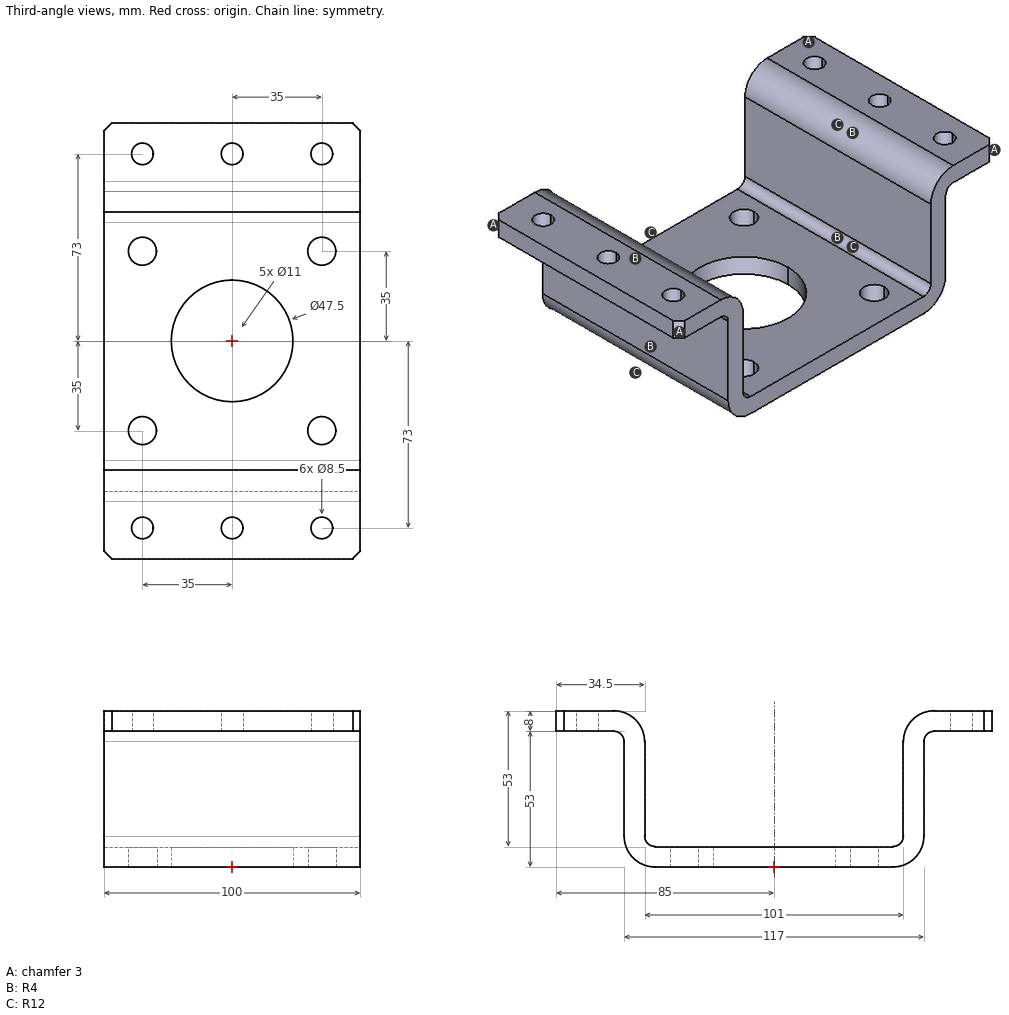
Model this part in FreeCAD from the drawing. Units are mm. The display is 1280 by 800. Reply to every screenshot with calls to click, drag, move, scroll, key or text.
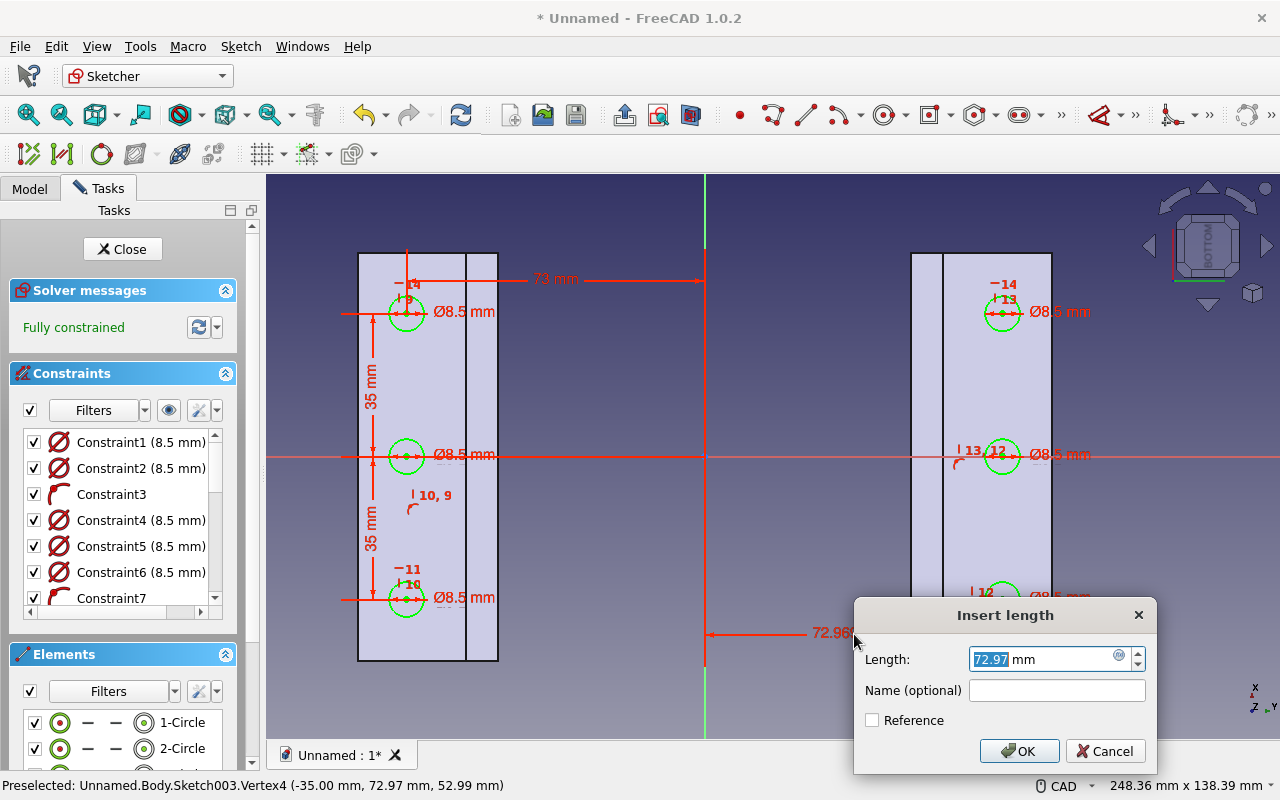
text(73)
key(Return)
key(Escape)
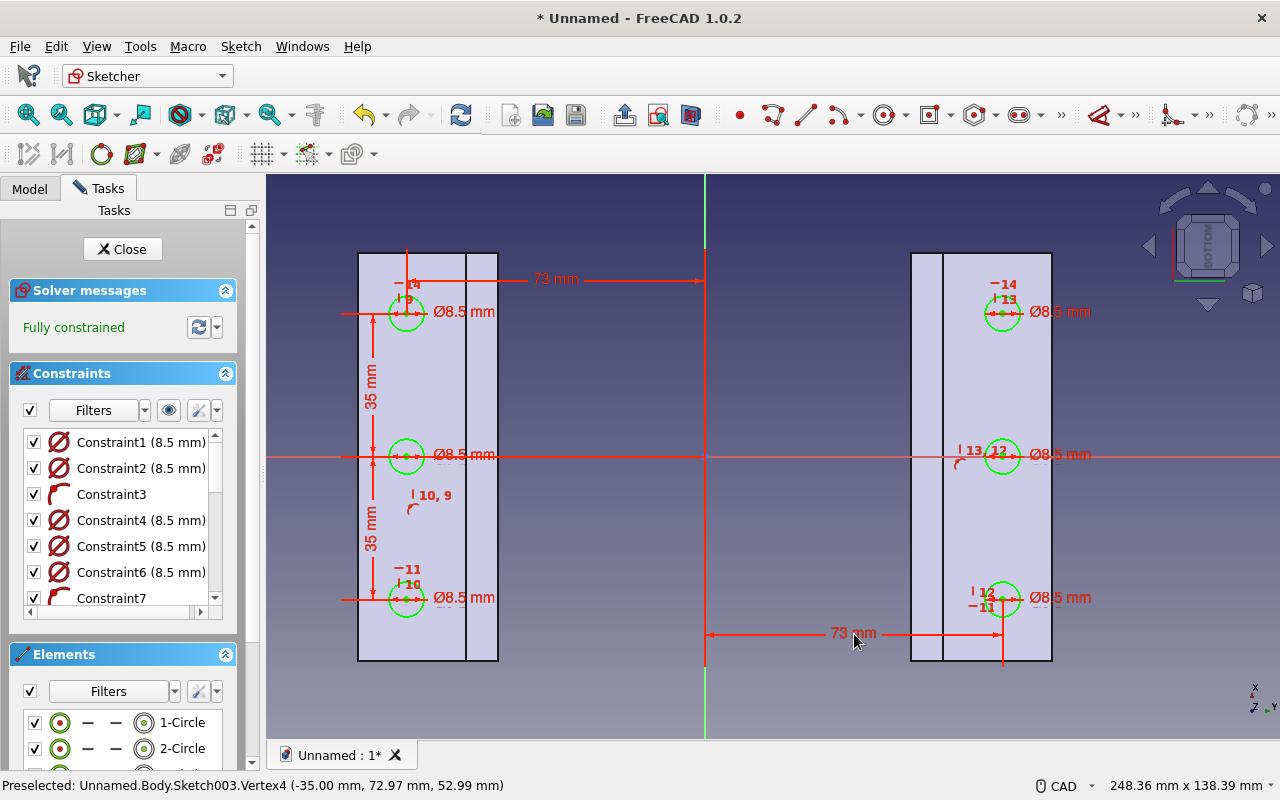
click(123, 249)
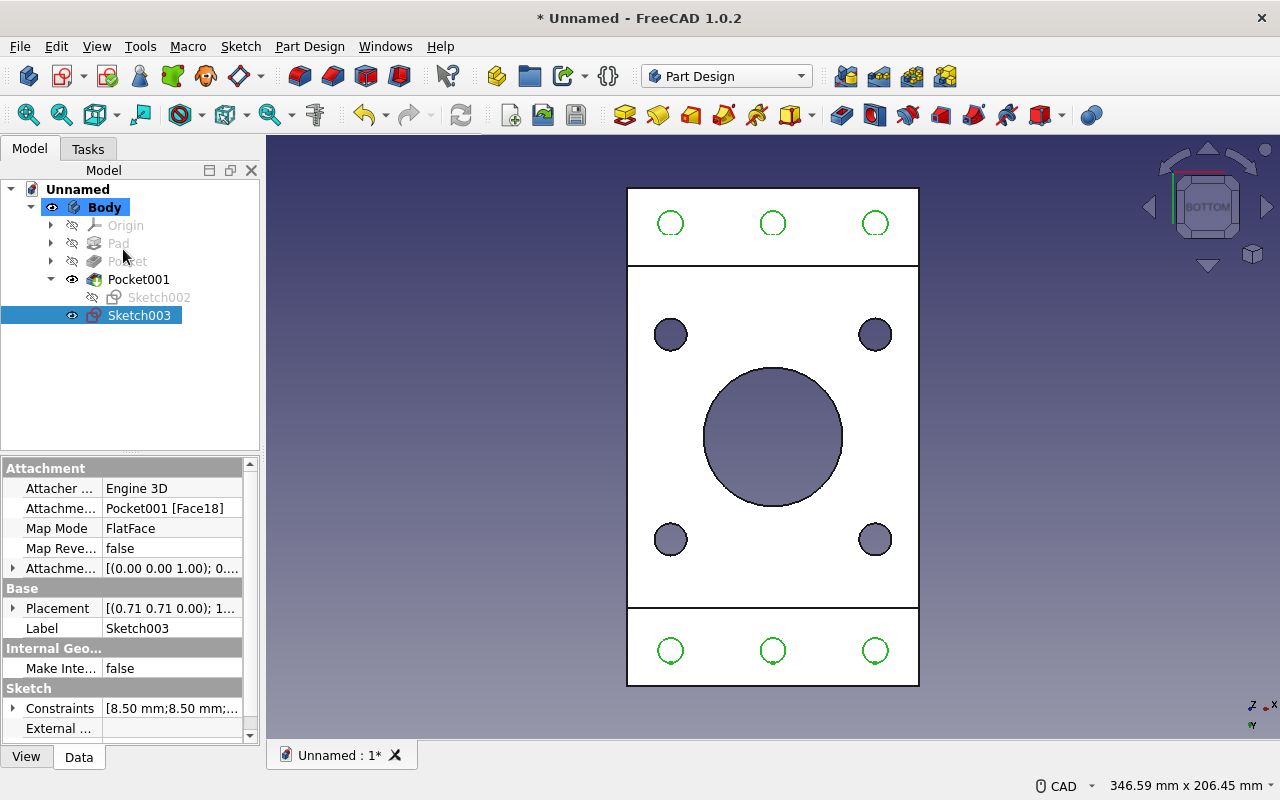
click(842, 116)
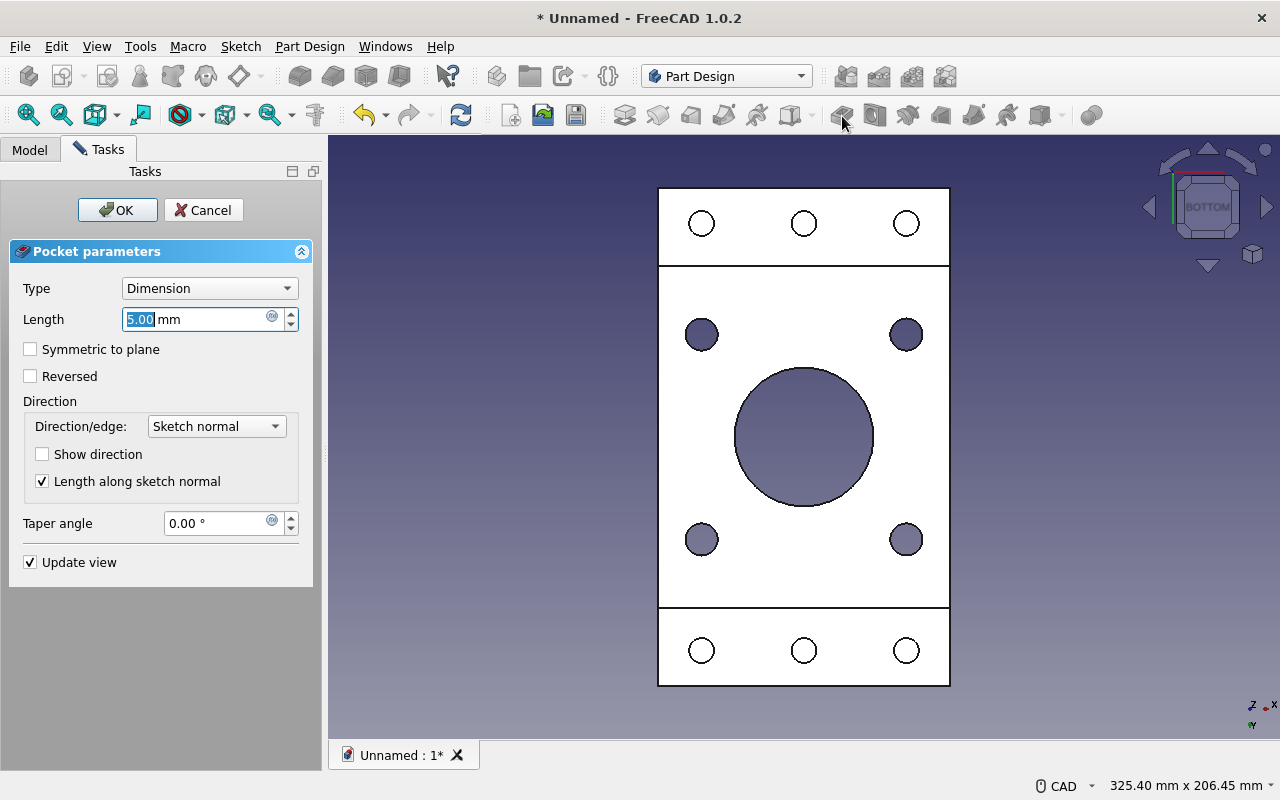
click(210, 288)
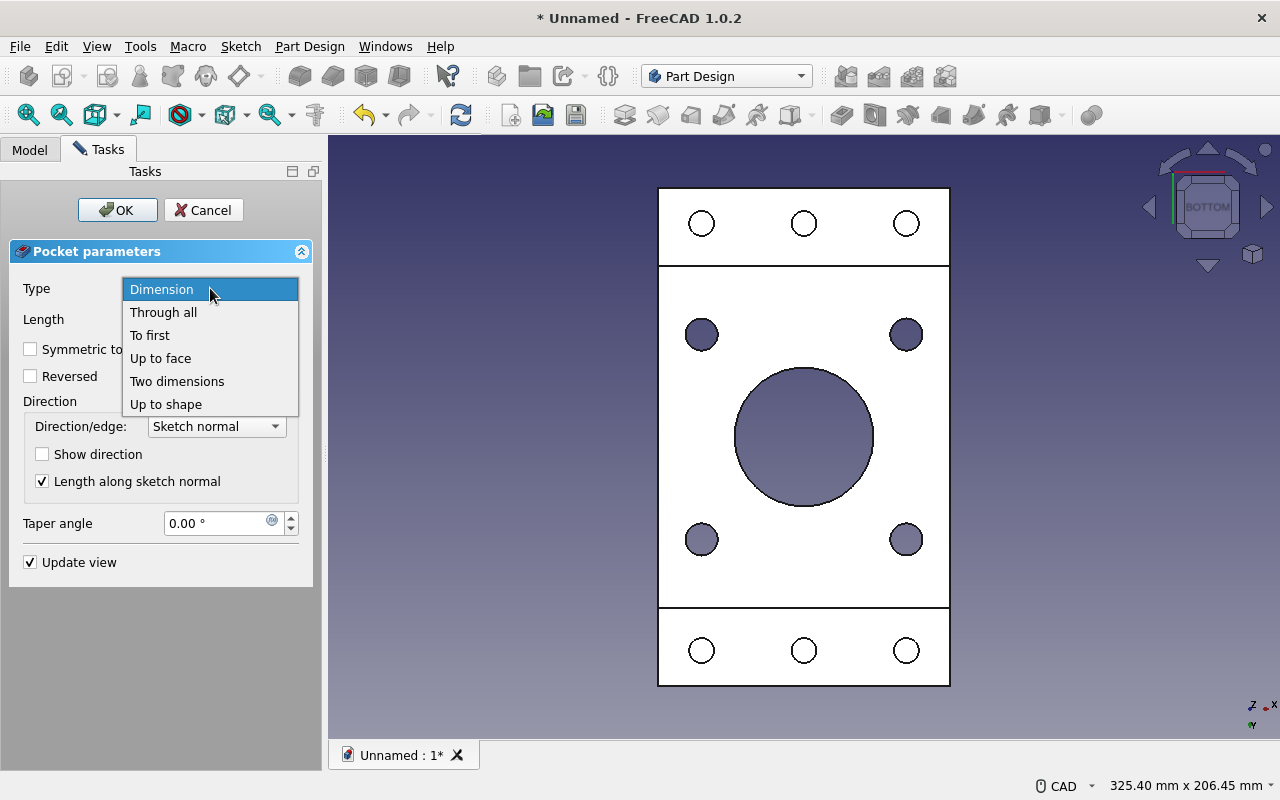
click(208, 312)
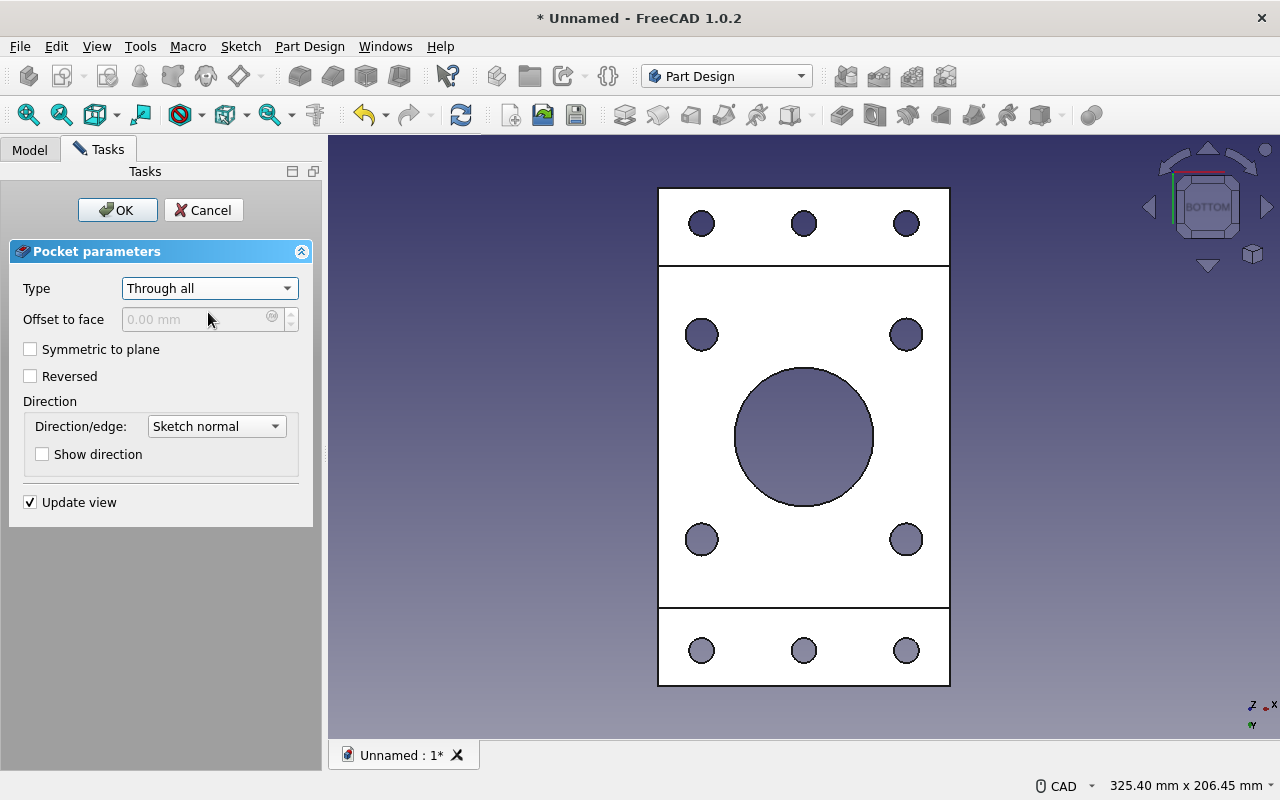
click(118, 210)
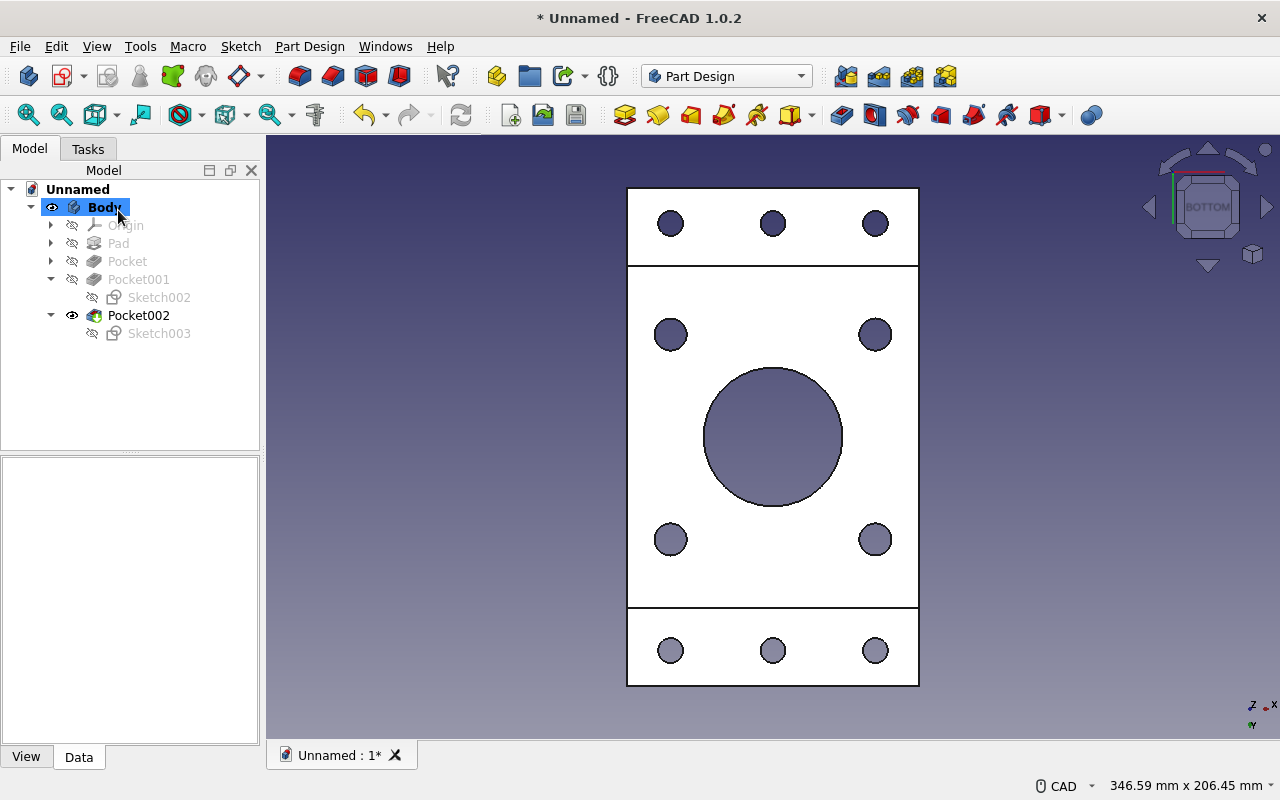
key(0)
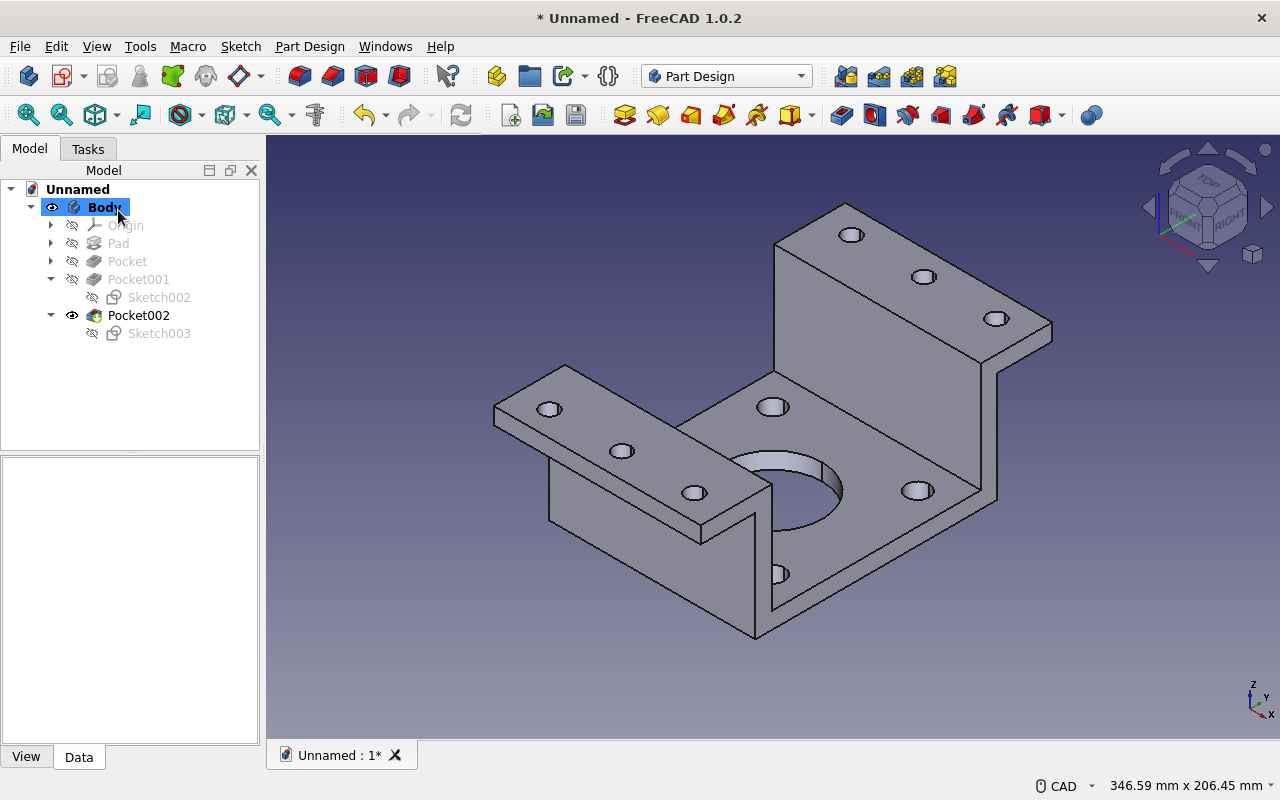
click(701, 534)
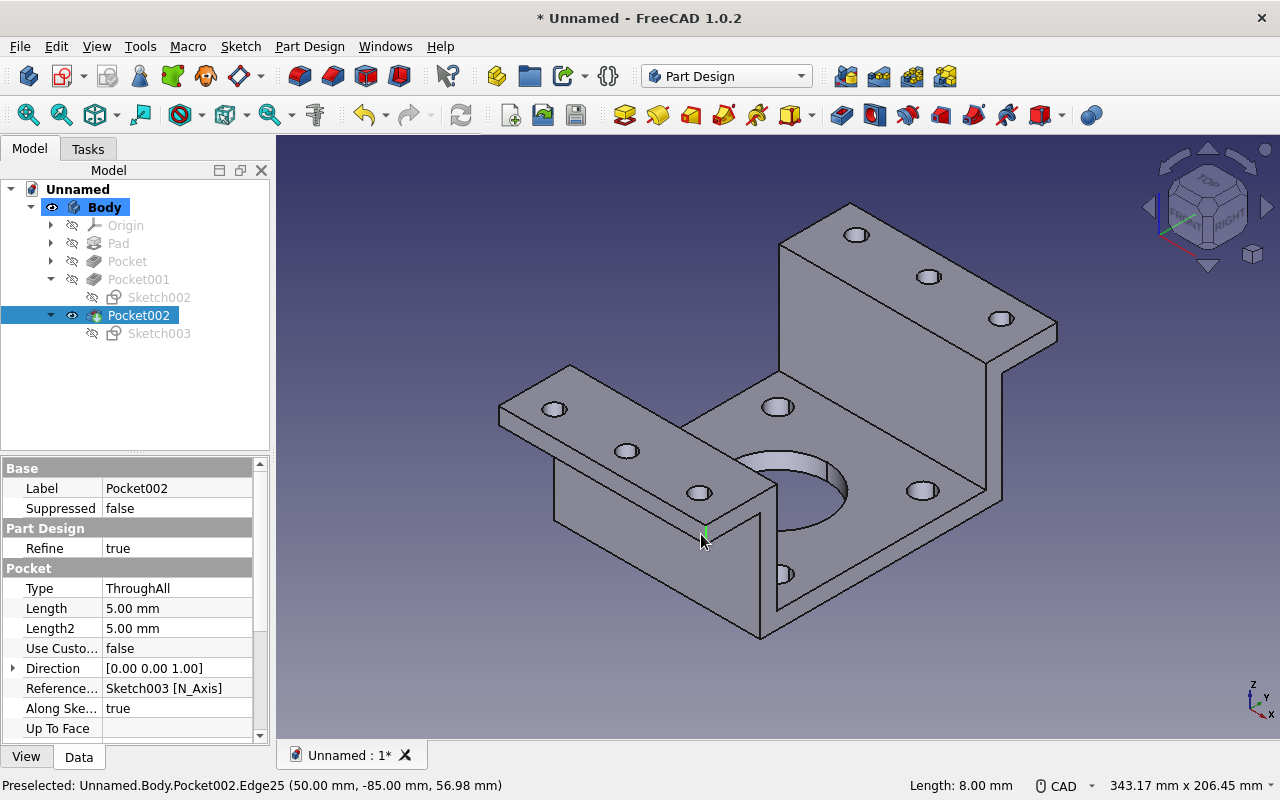
key(2)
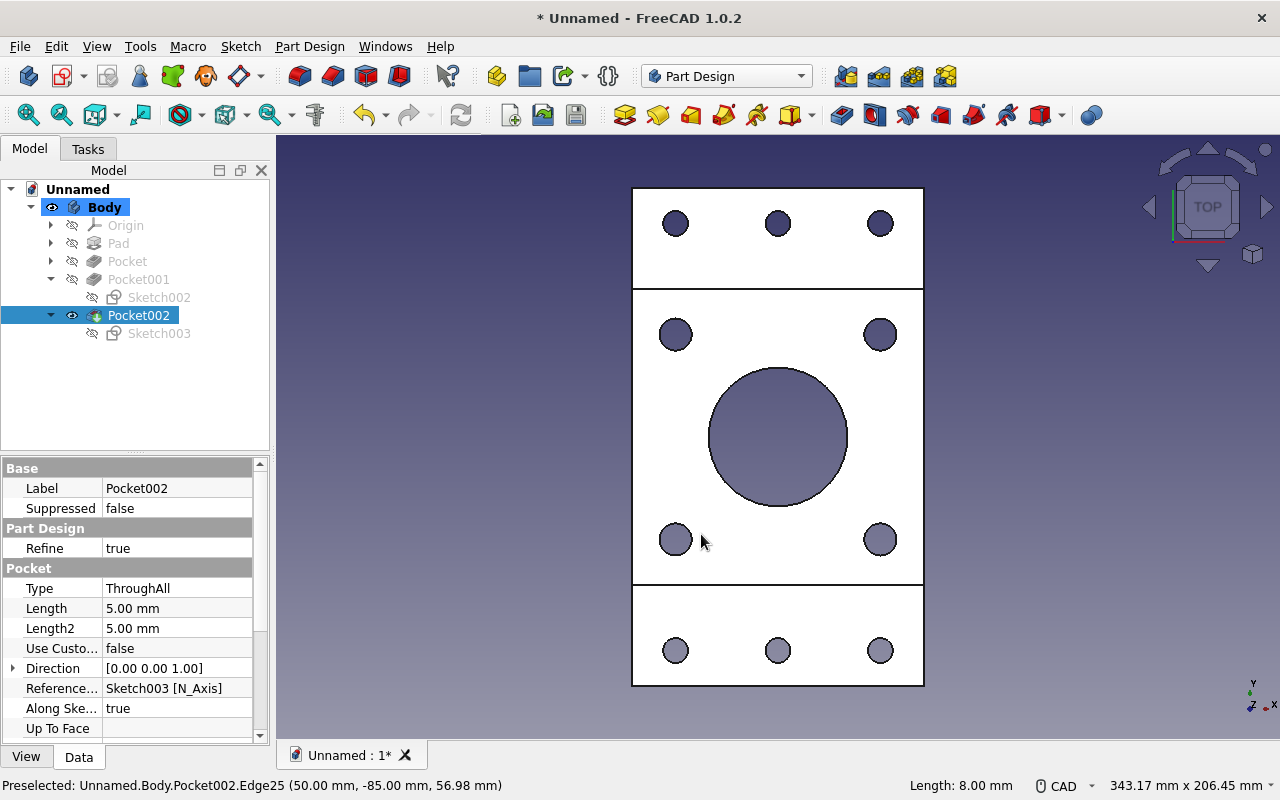
key(1)